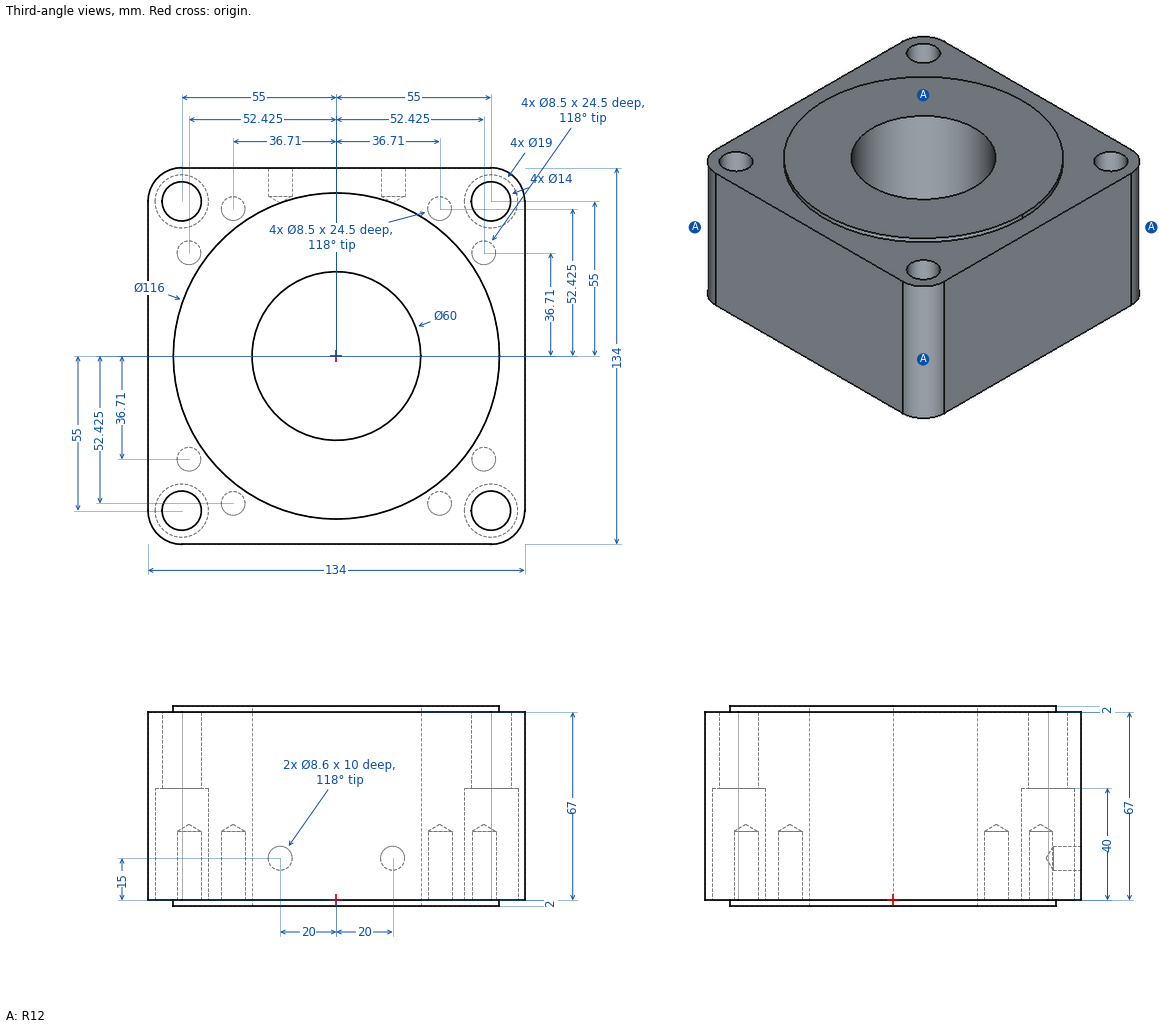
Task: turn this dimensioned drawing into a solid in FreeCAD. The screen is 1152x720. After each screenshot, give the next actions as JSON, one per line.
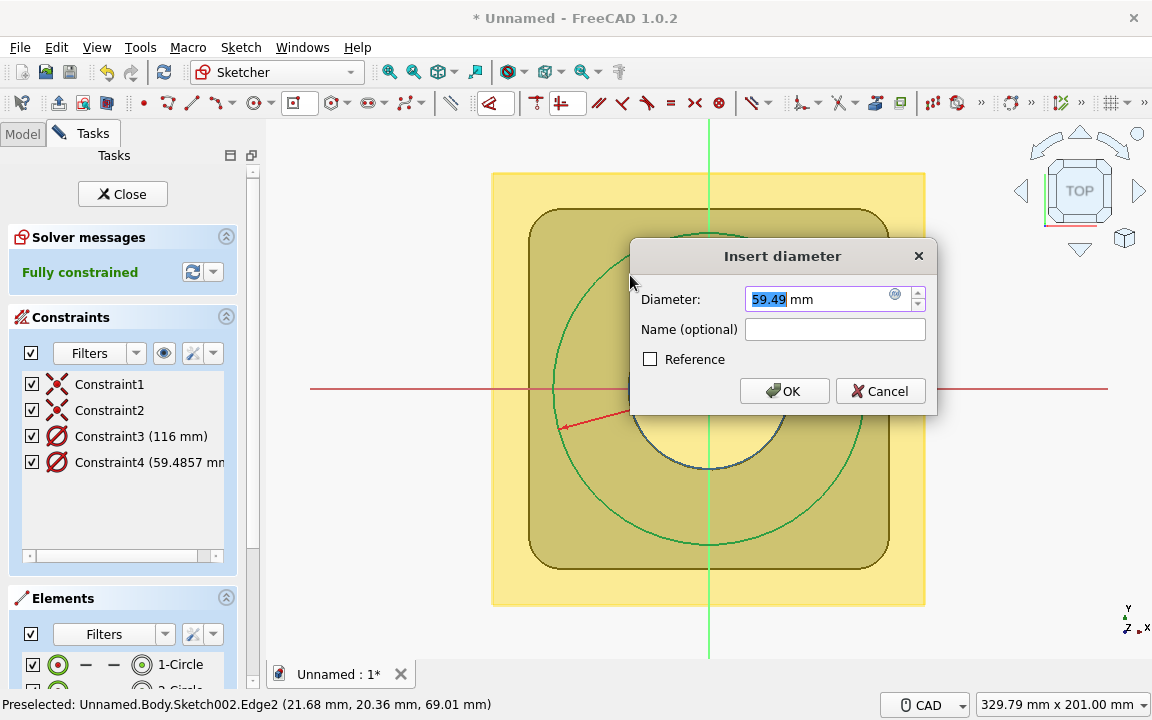
{"action": "type", "text": "60"}
{"action": "key", "text": "Return"}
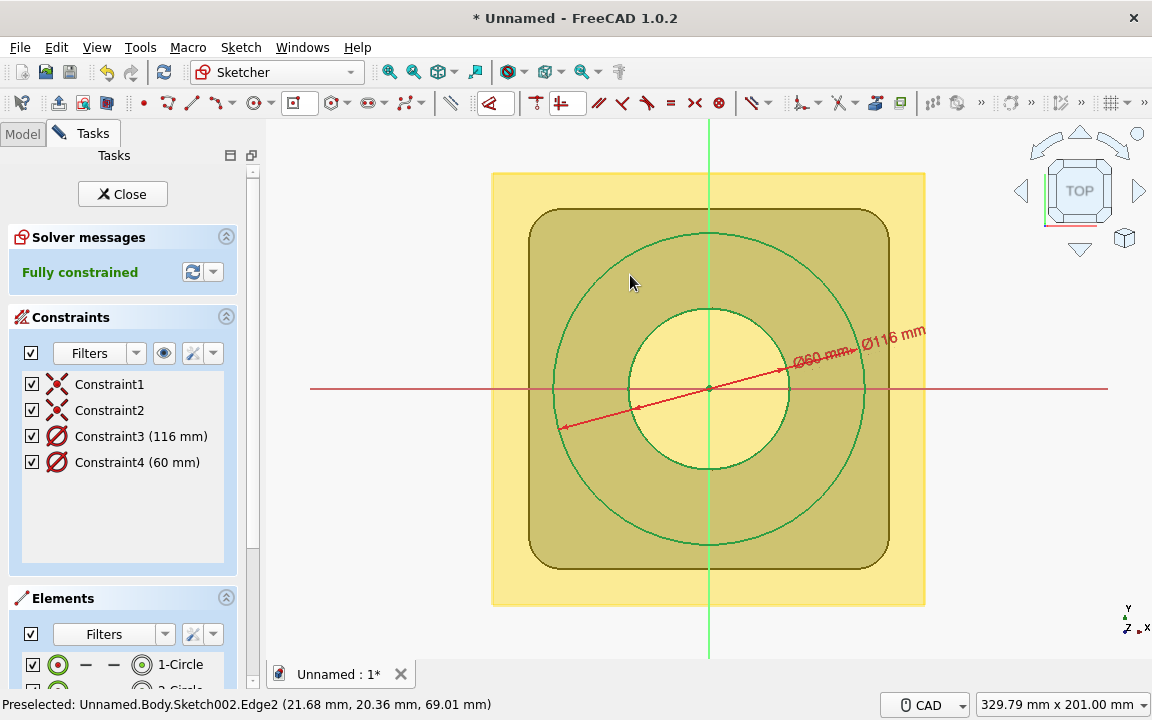
{"action": "left_click", "coordinate": [123, 194]}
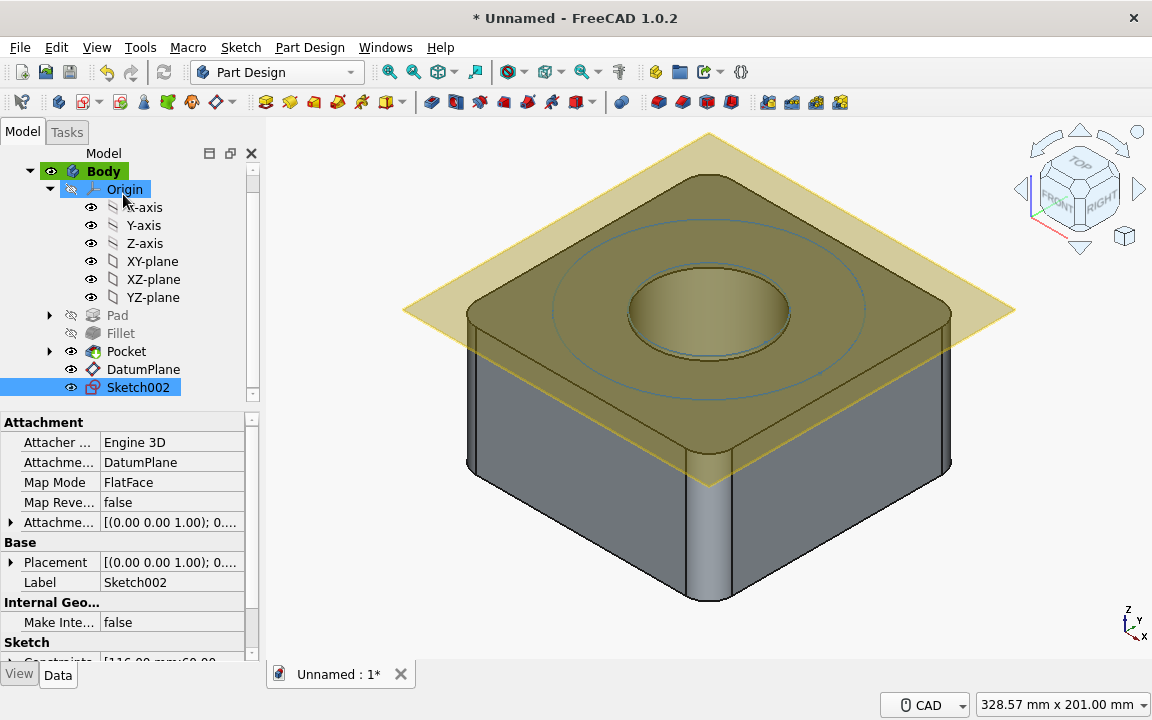
{"action": "left_click", "coordinate": [266, 102]}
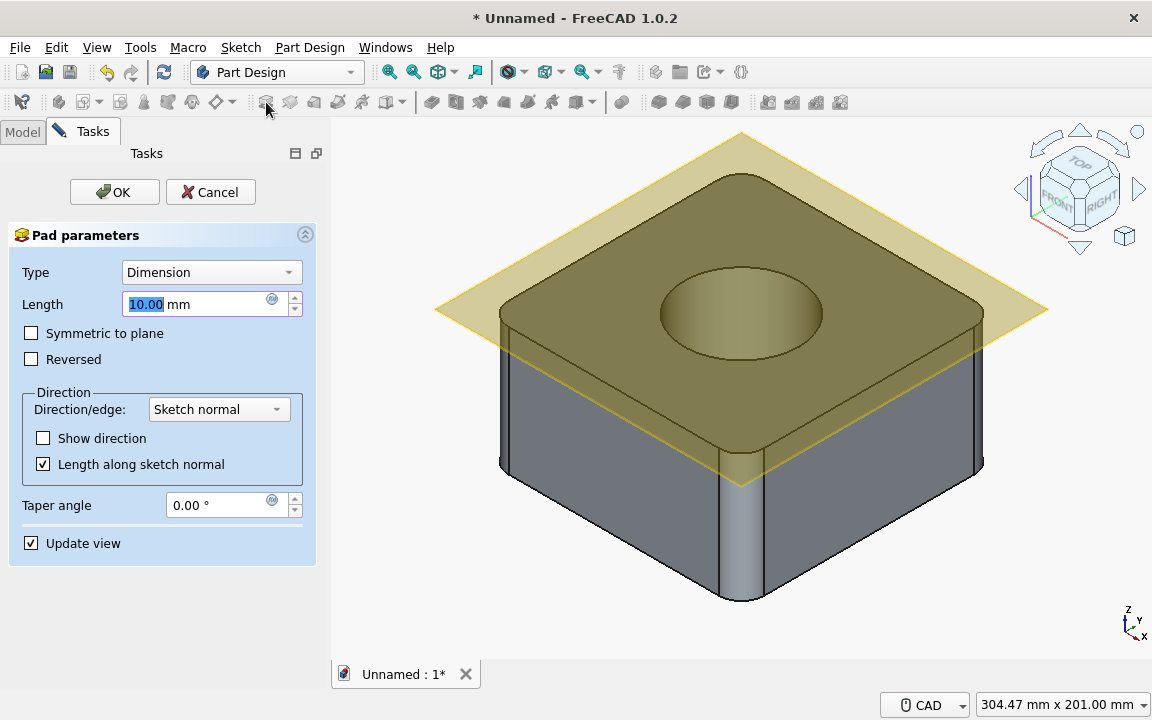
{"action": "type", "text": "2"}
{"action": "key", "text": "Tab"}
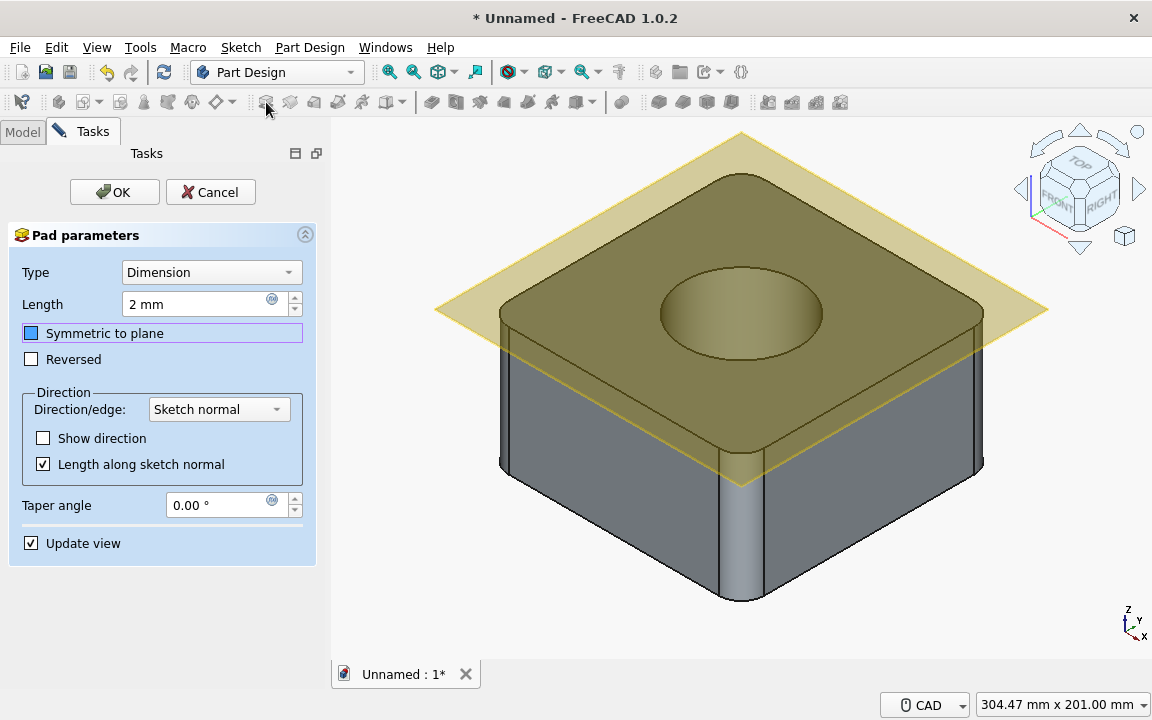
{"action": "left_click", "coordinate": [30, 359]}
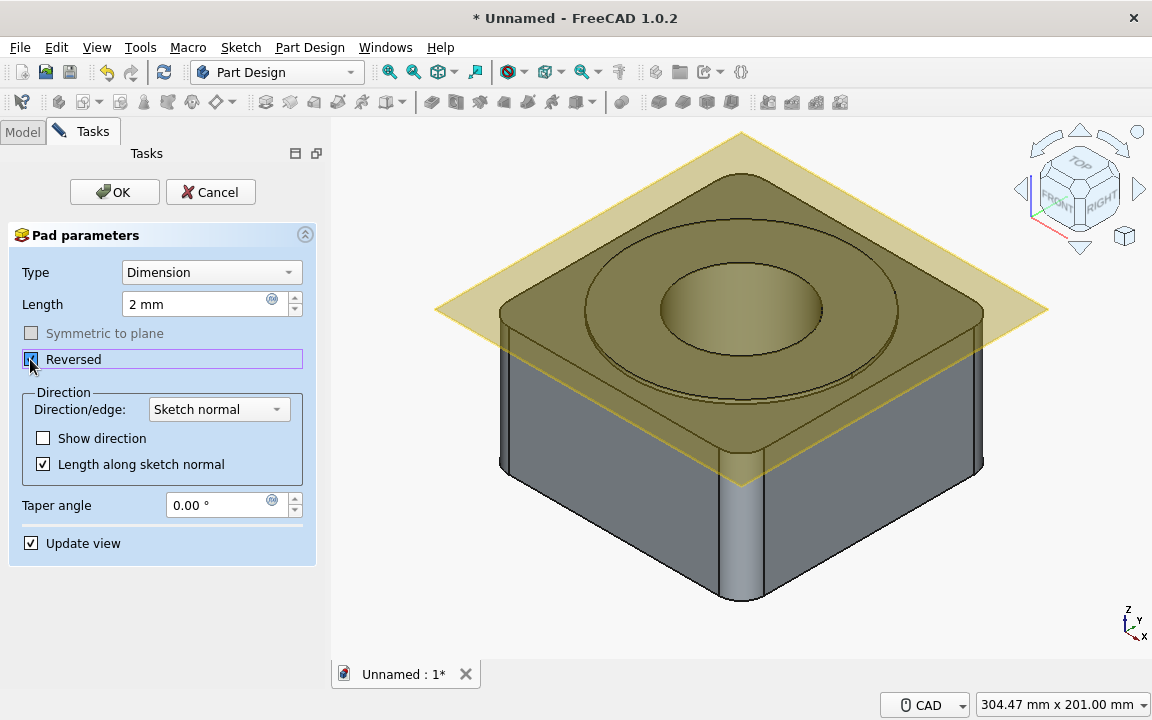
{"action": "left_click", "coordinate": [115, 192]}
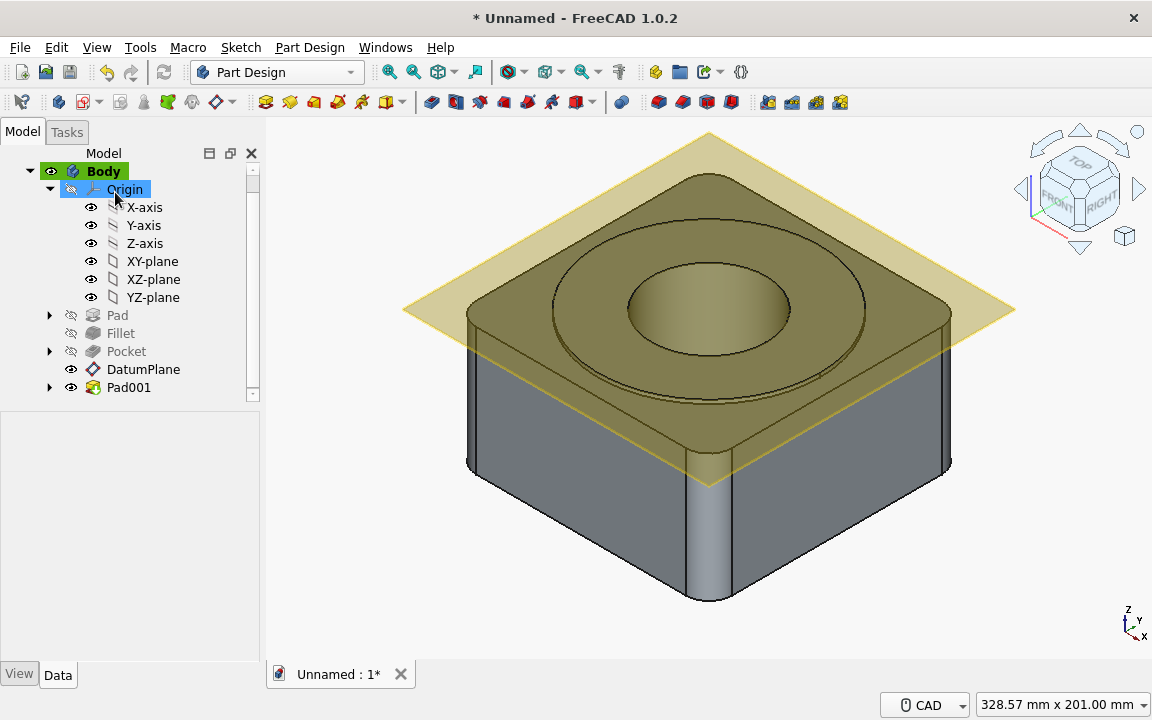
{"action": "left_click", "coordinate": [116, 369]}
{"action": "key", "text": "space"}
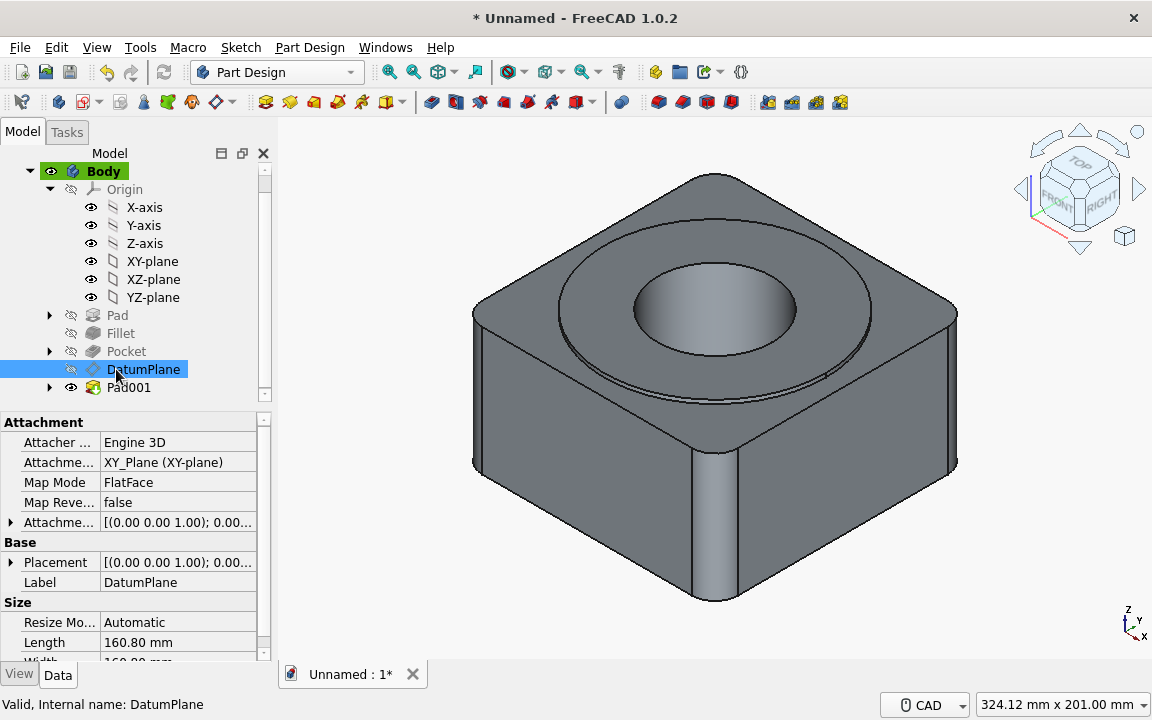
{"action": "key", "text": "5"}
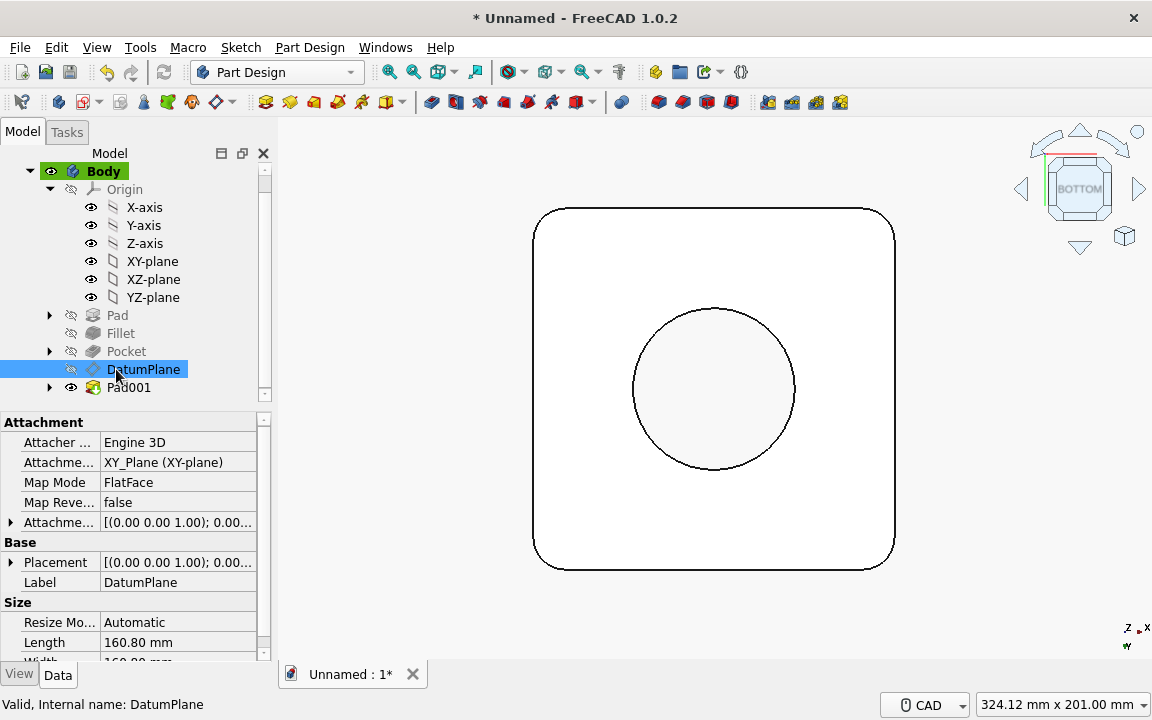
{"action": "left_click", "coordinate": [817, 491]}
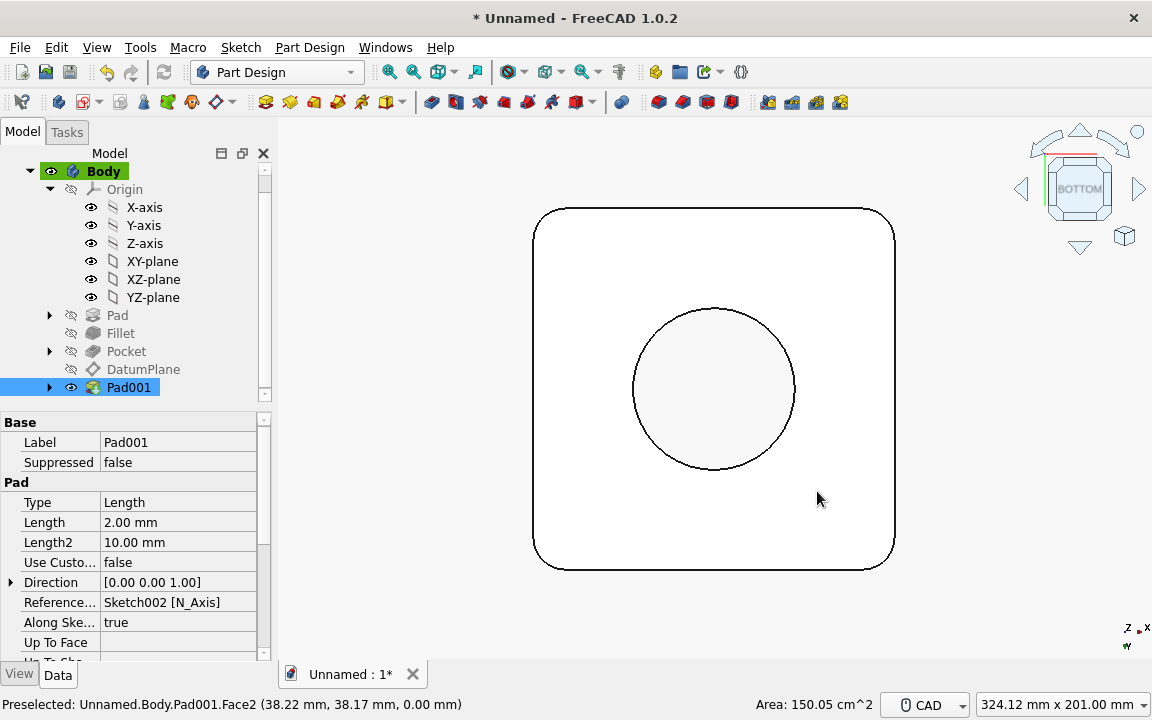
{"action": "left_click", "coordinate": [84, 102]}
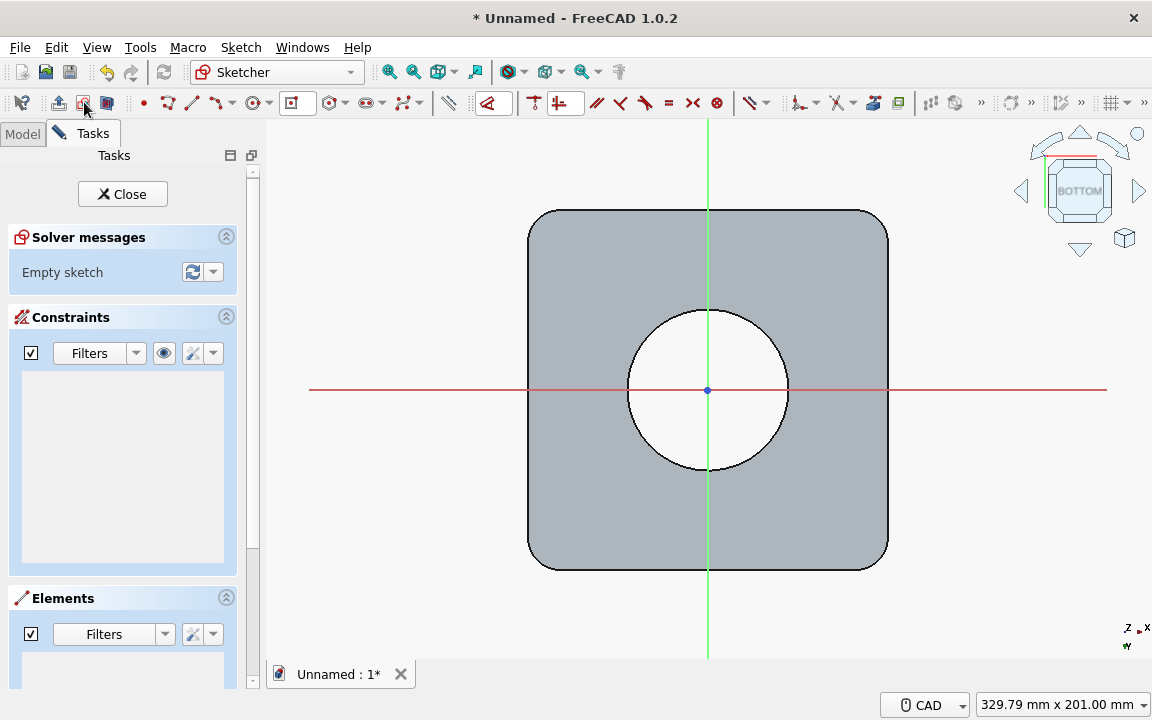
{"action": "left_click", "coordinate": [254, 104]}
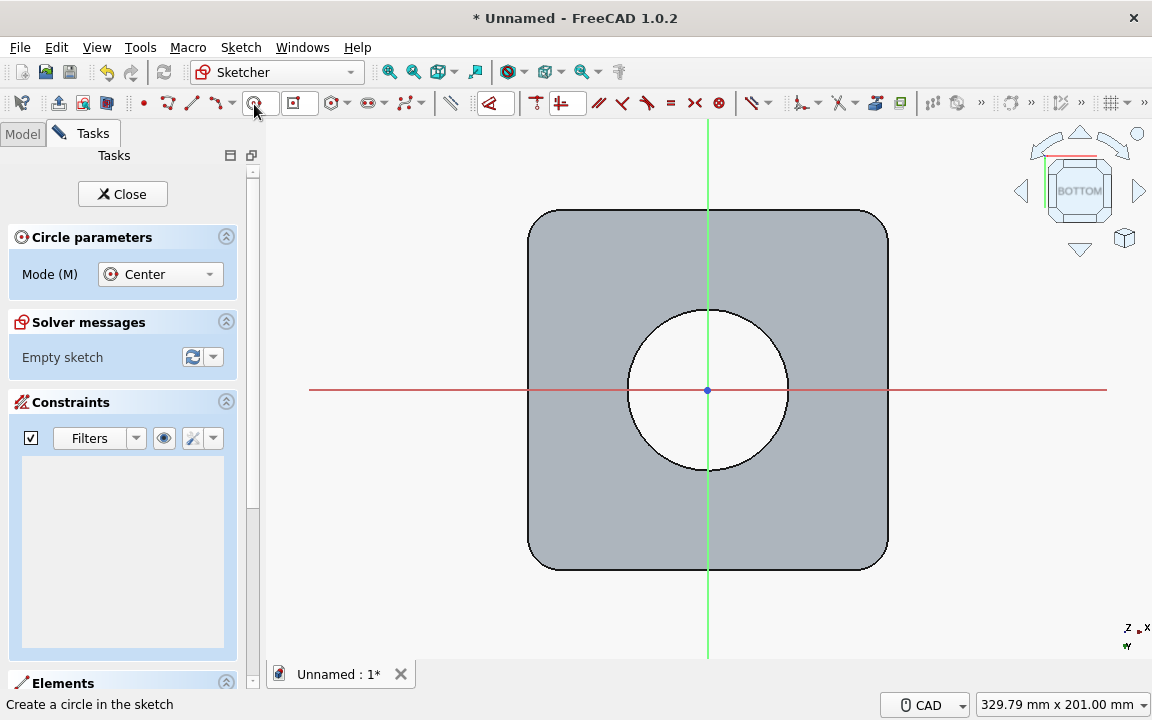
{"action": "left_click", "coordinate": [708, 390]}
{"action": "left_click", "coordinate": [818, 280]}